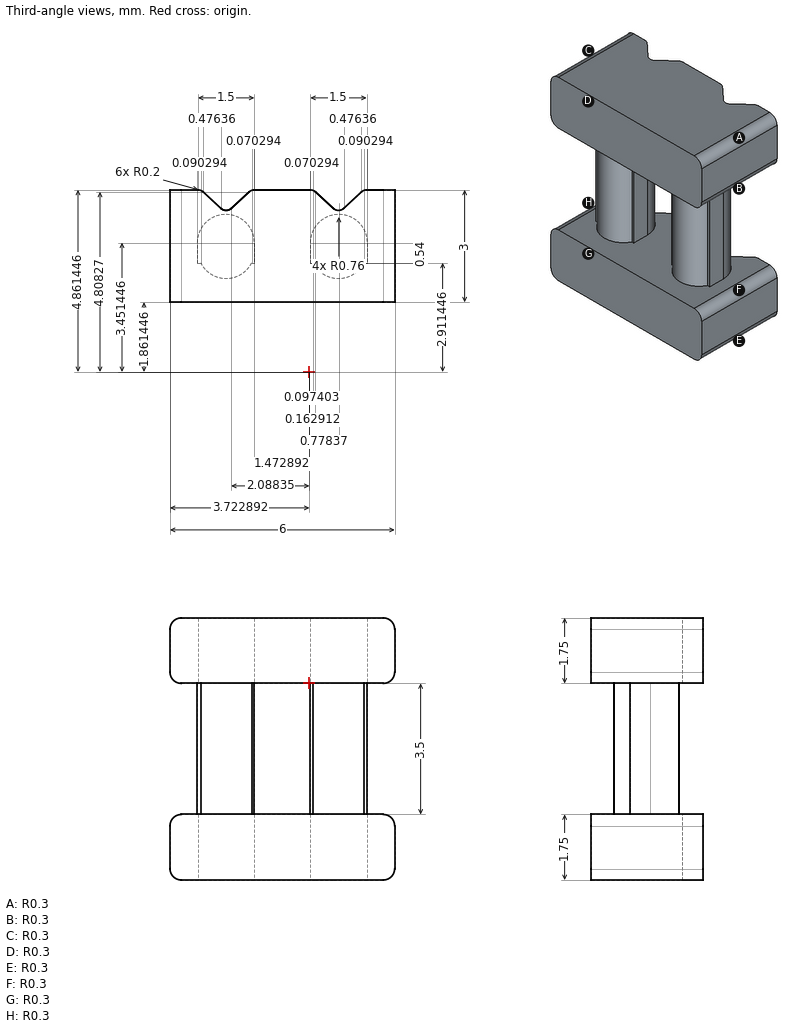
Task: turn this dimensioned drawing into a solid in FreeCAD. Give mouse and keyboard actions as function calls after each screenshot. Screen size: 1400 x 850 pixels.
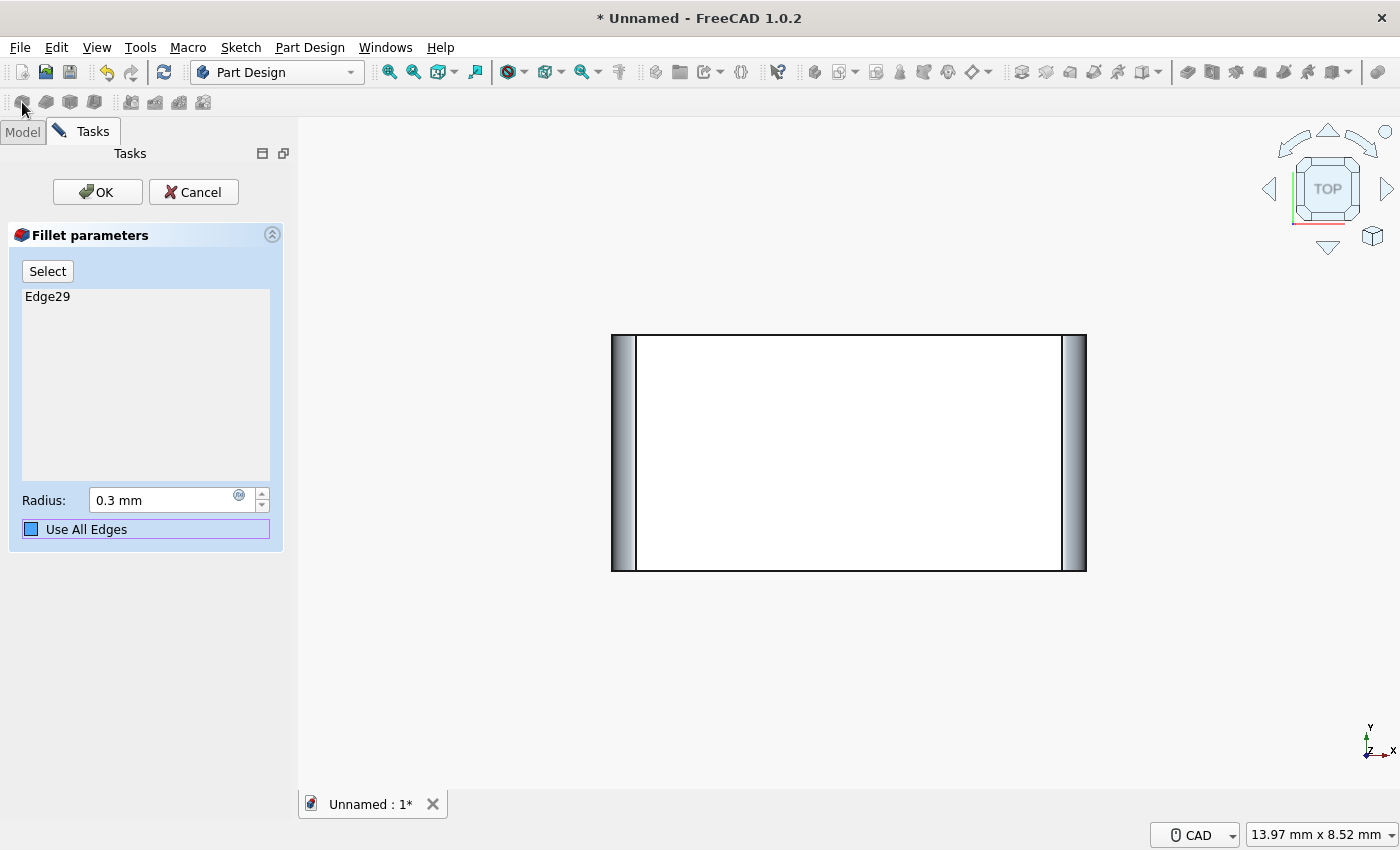
click(98, 192)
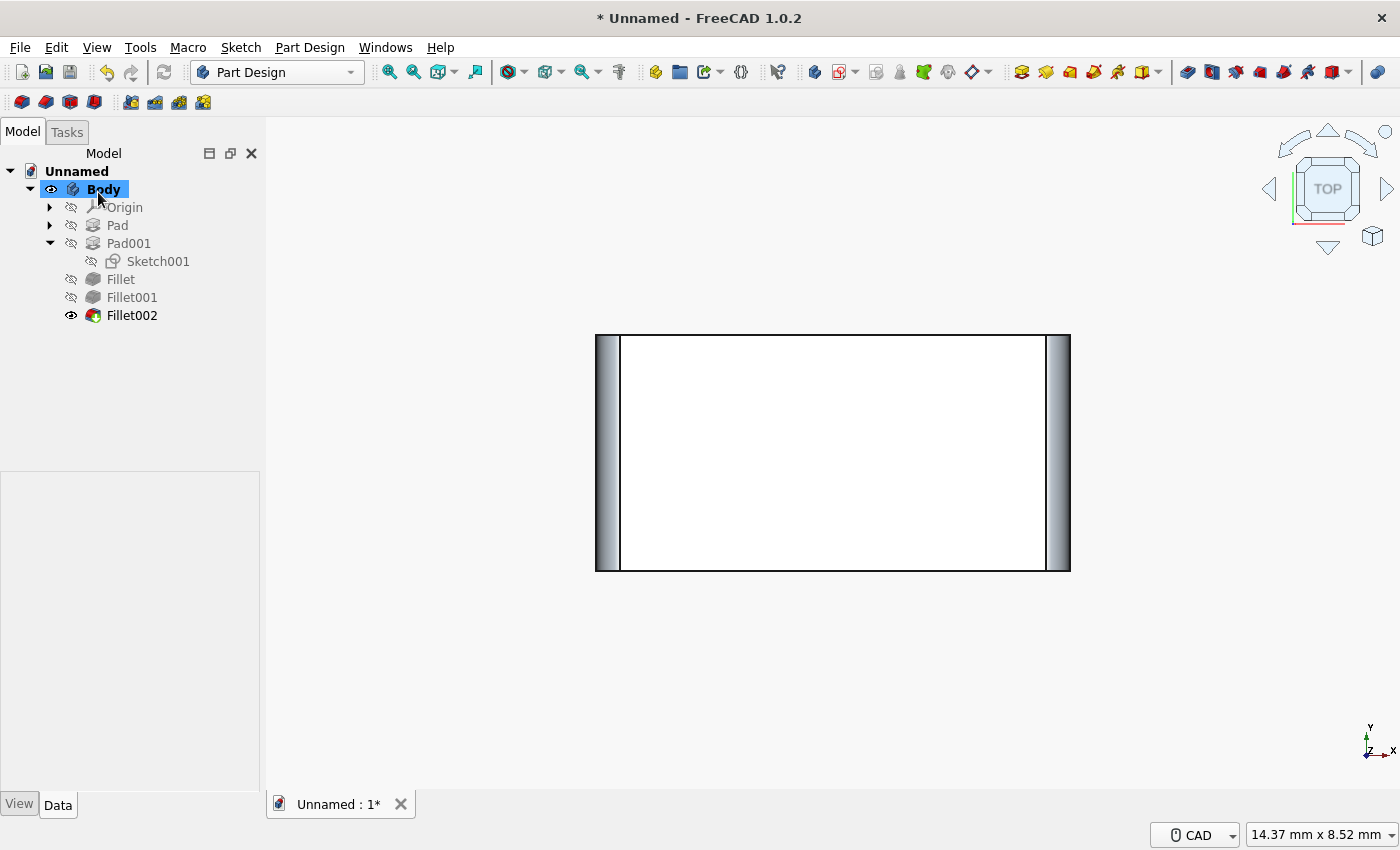
key(v)
key(f)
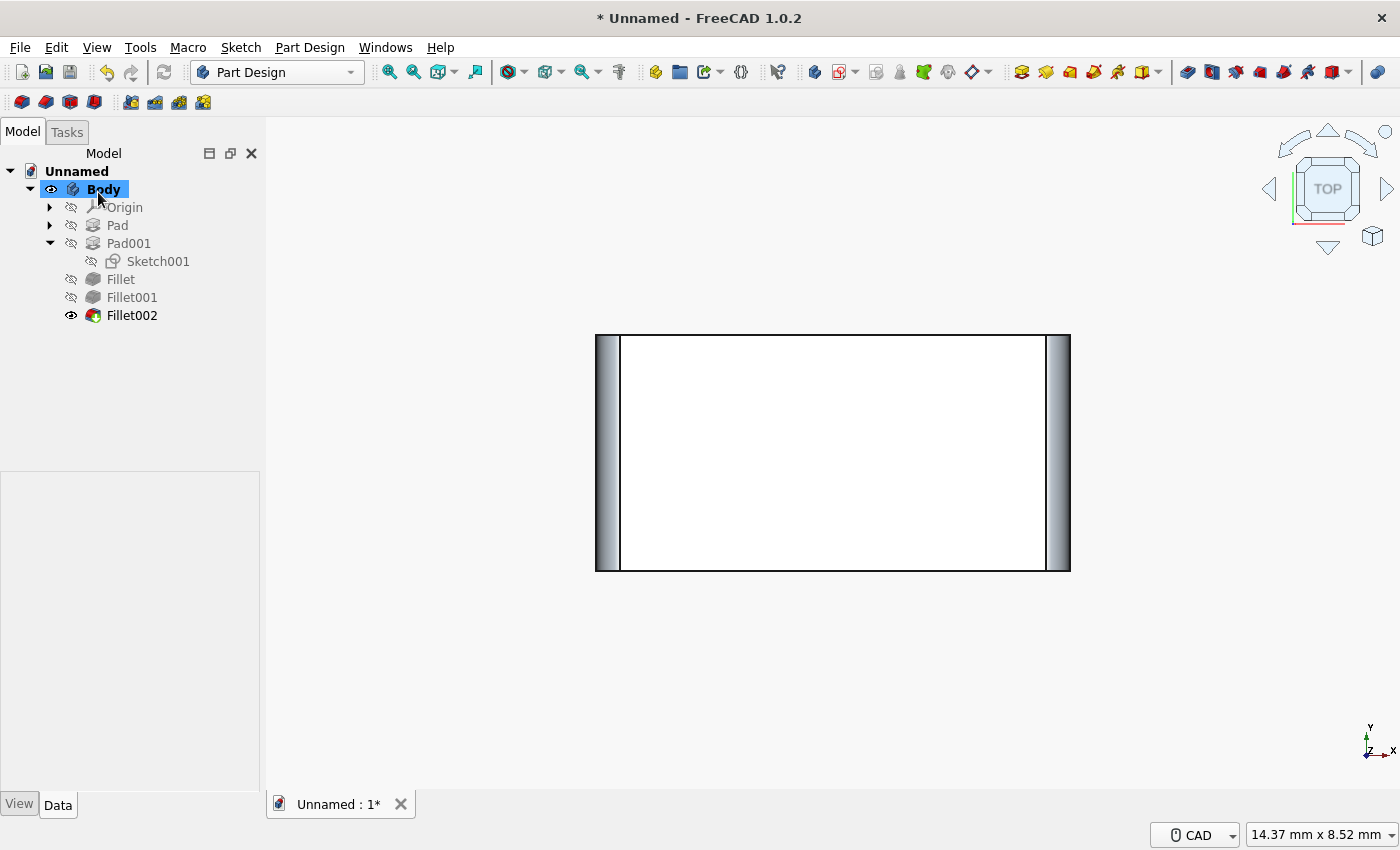
key(0)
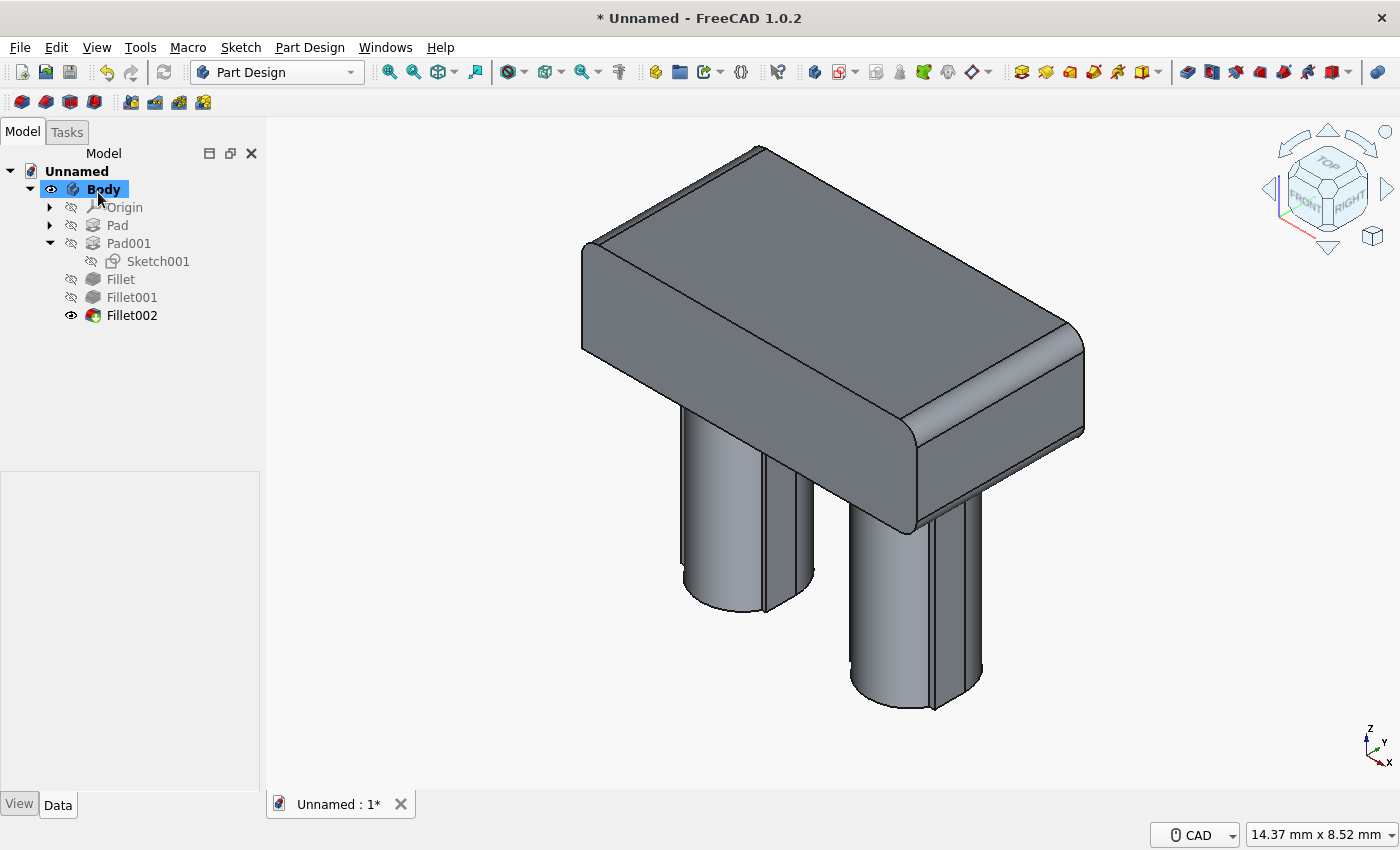
key(2)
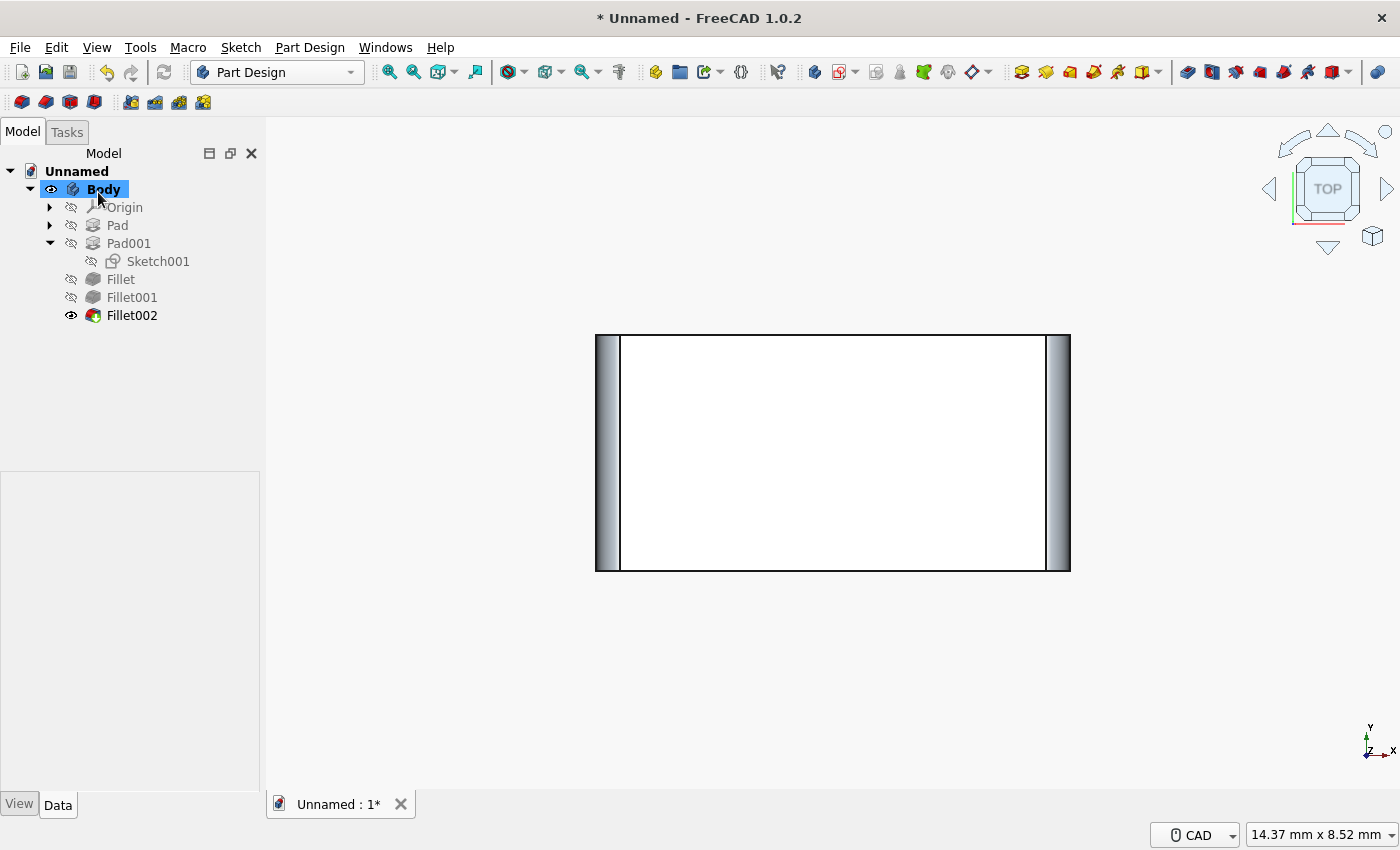
click(390, 72)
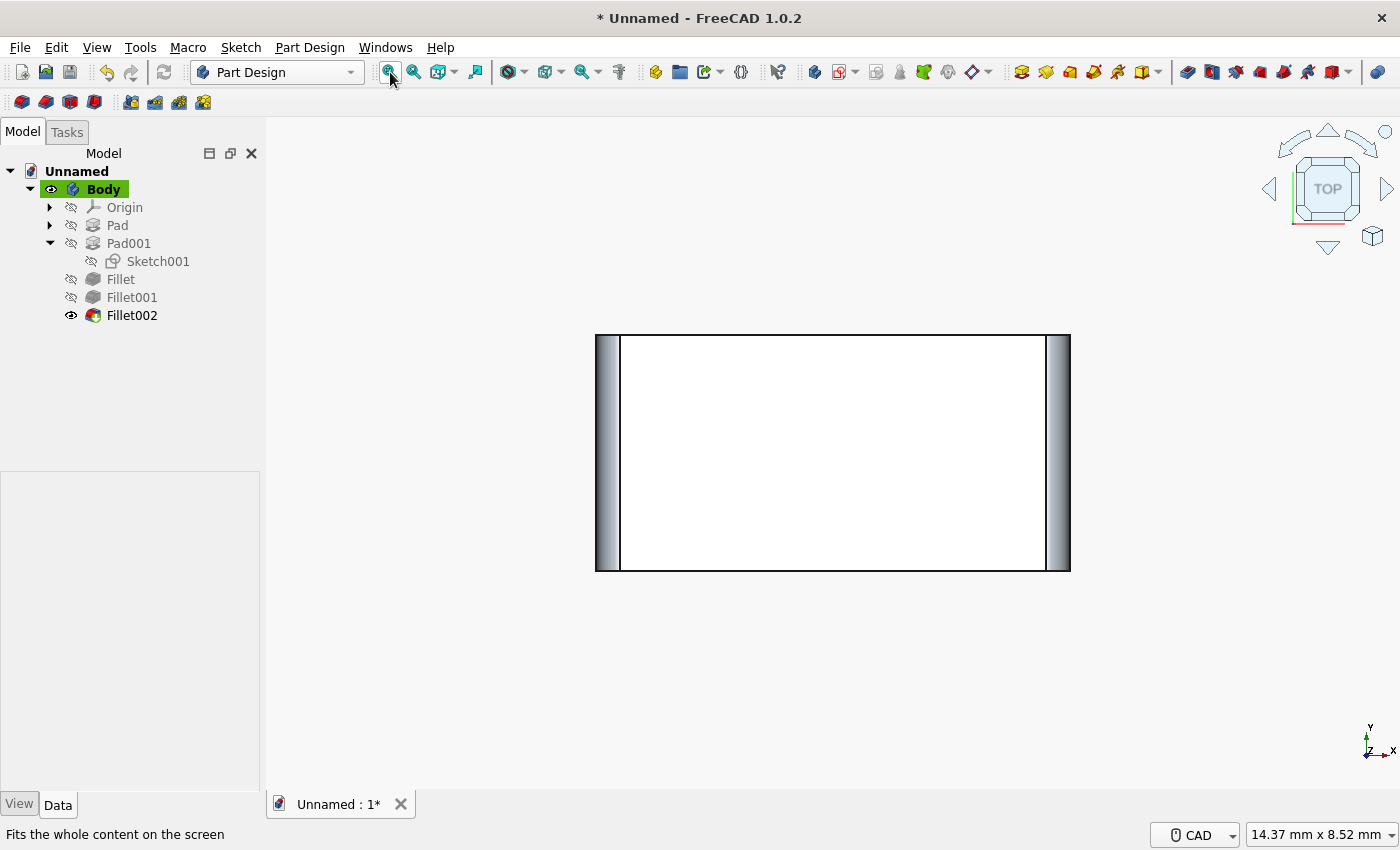
key(1)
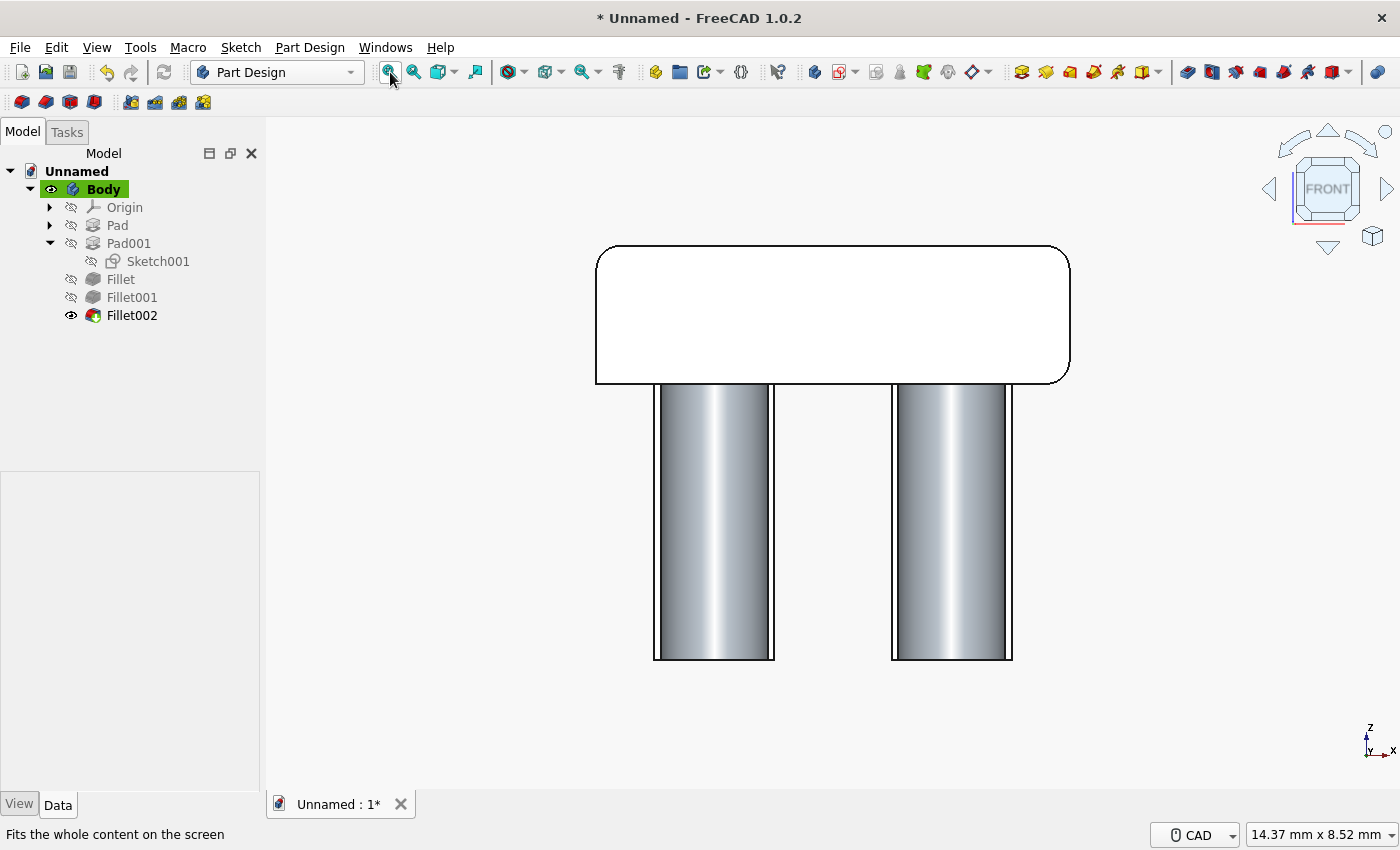
key(3)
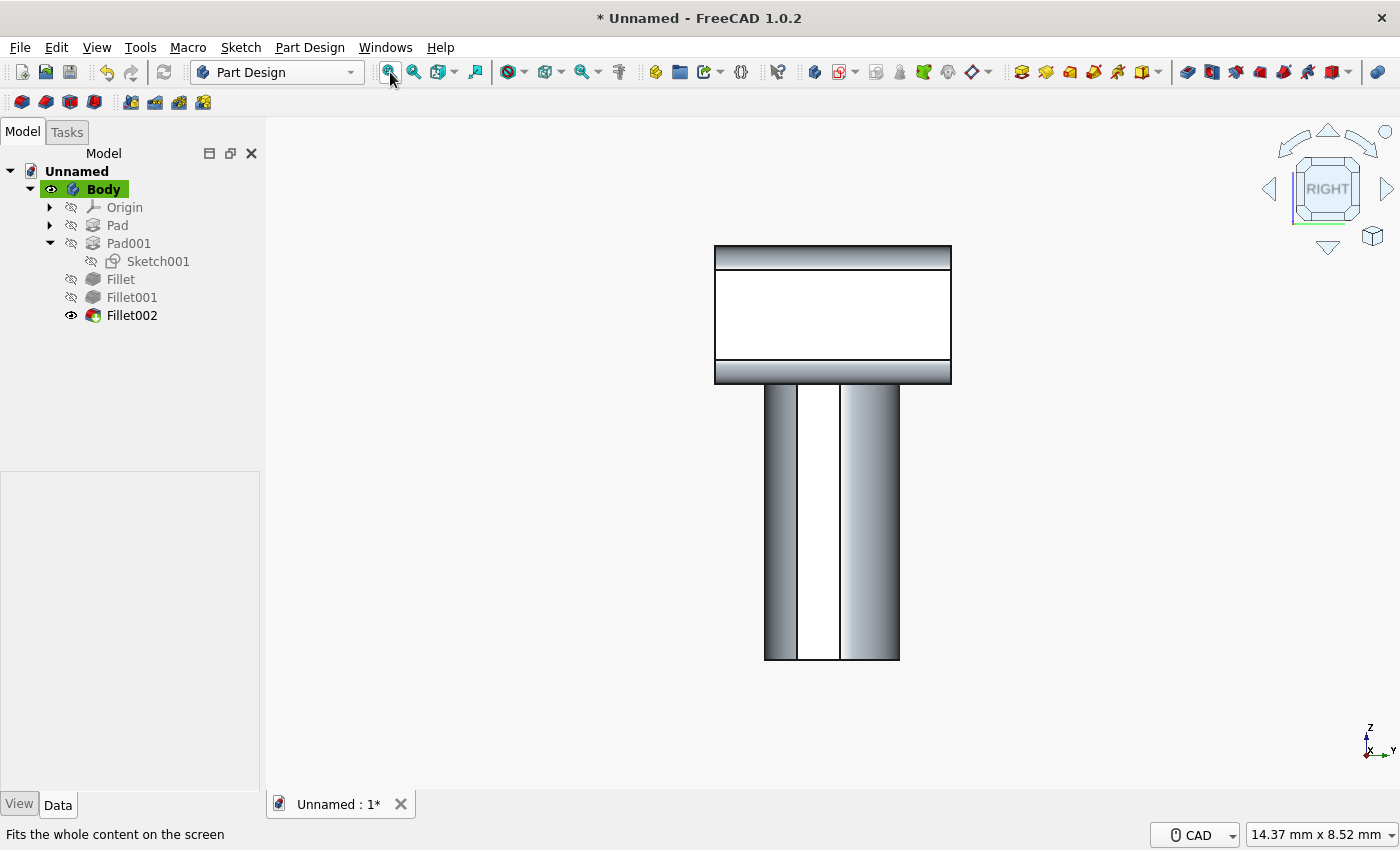
key(5)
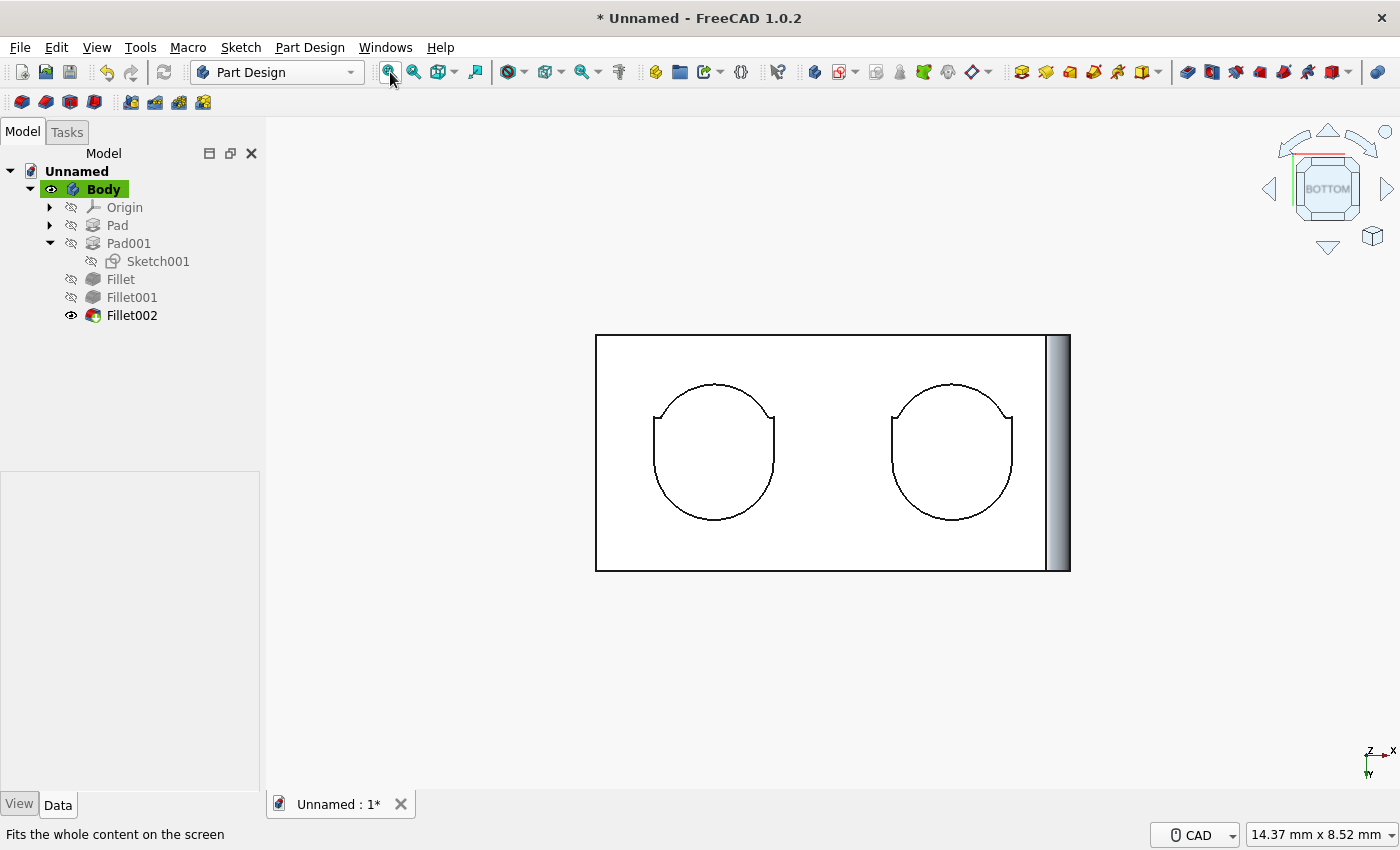
click(390, 72)